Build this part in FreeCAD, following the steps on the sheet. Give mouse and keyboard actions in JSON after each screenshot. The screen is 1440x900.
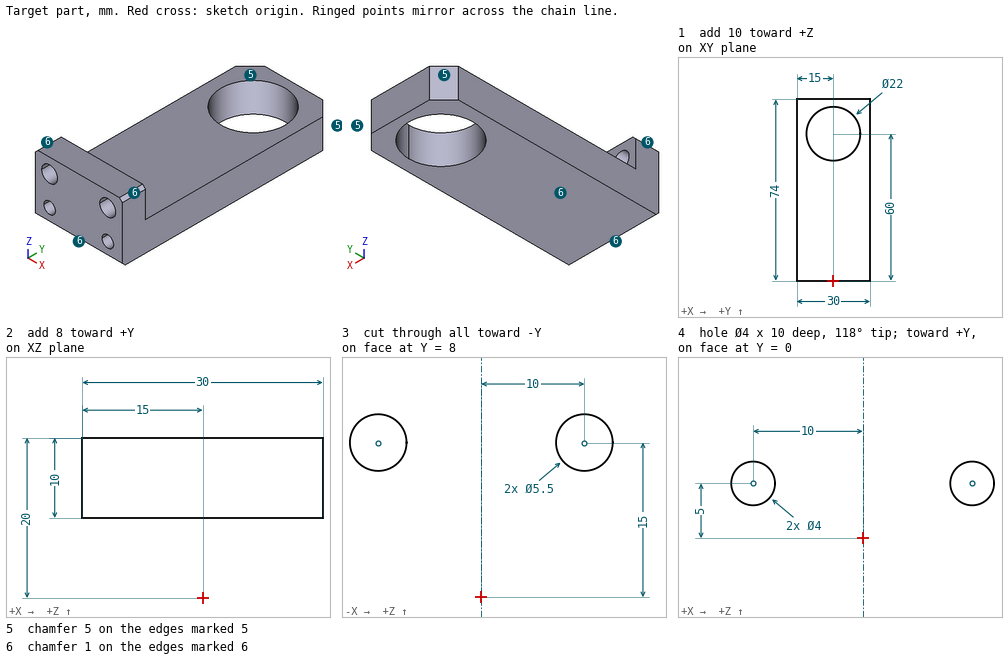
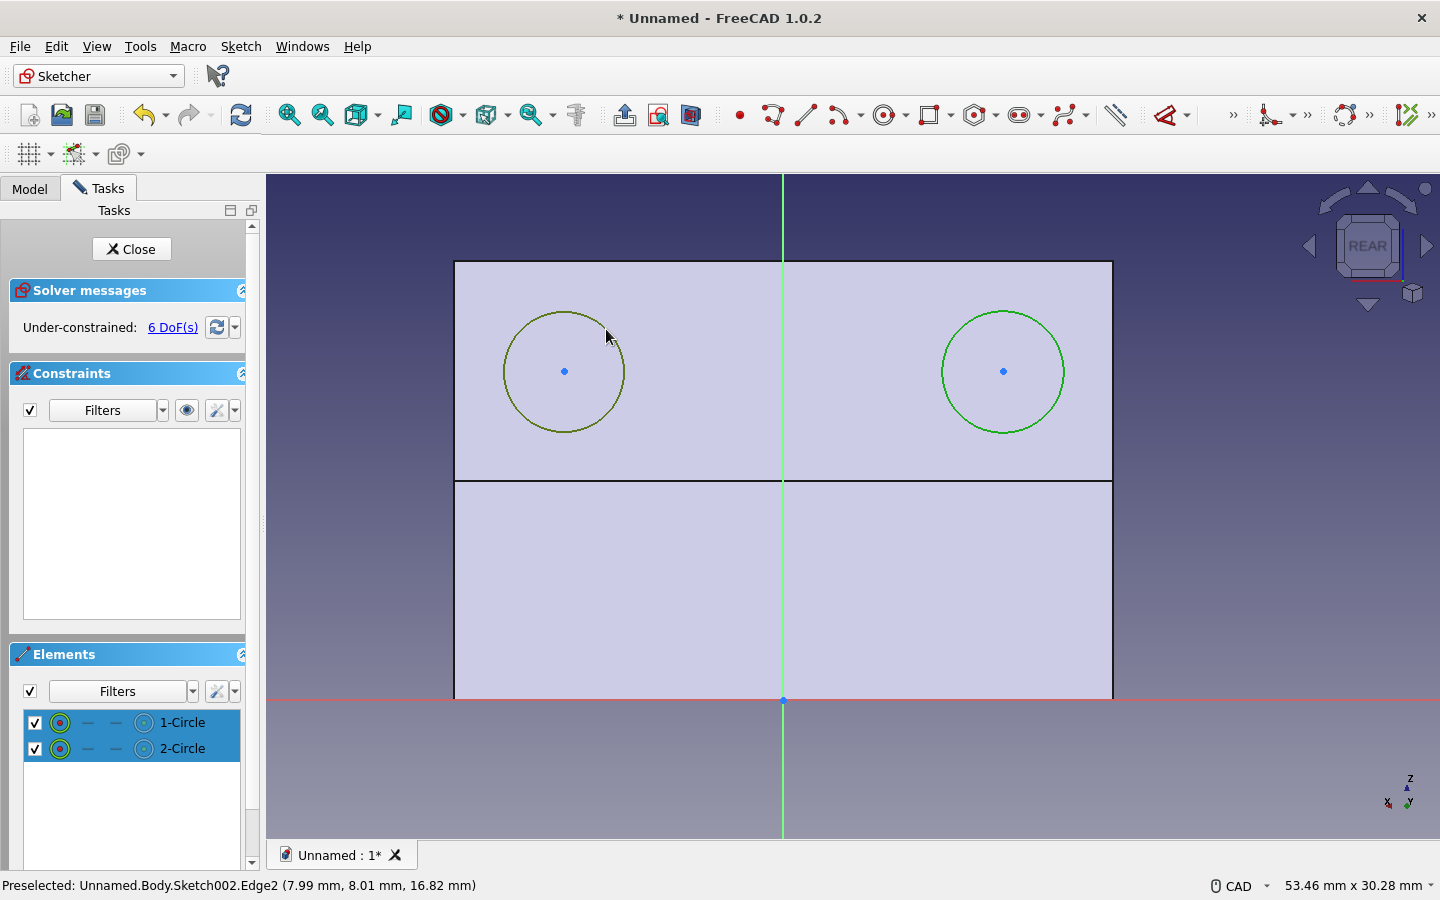
{"action": "key", "text": "e"}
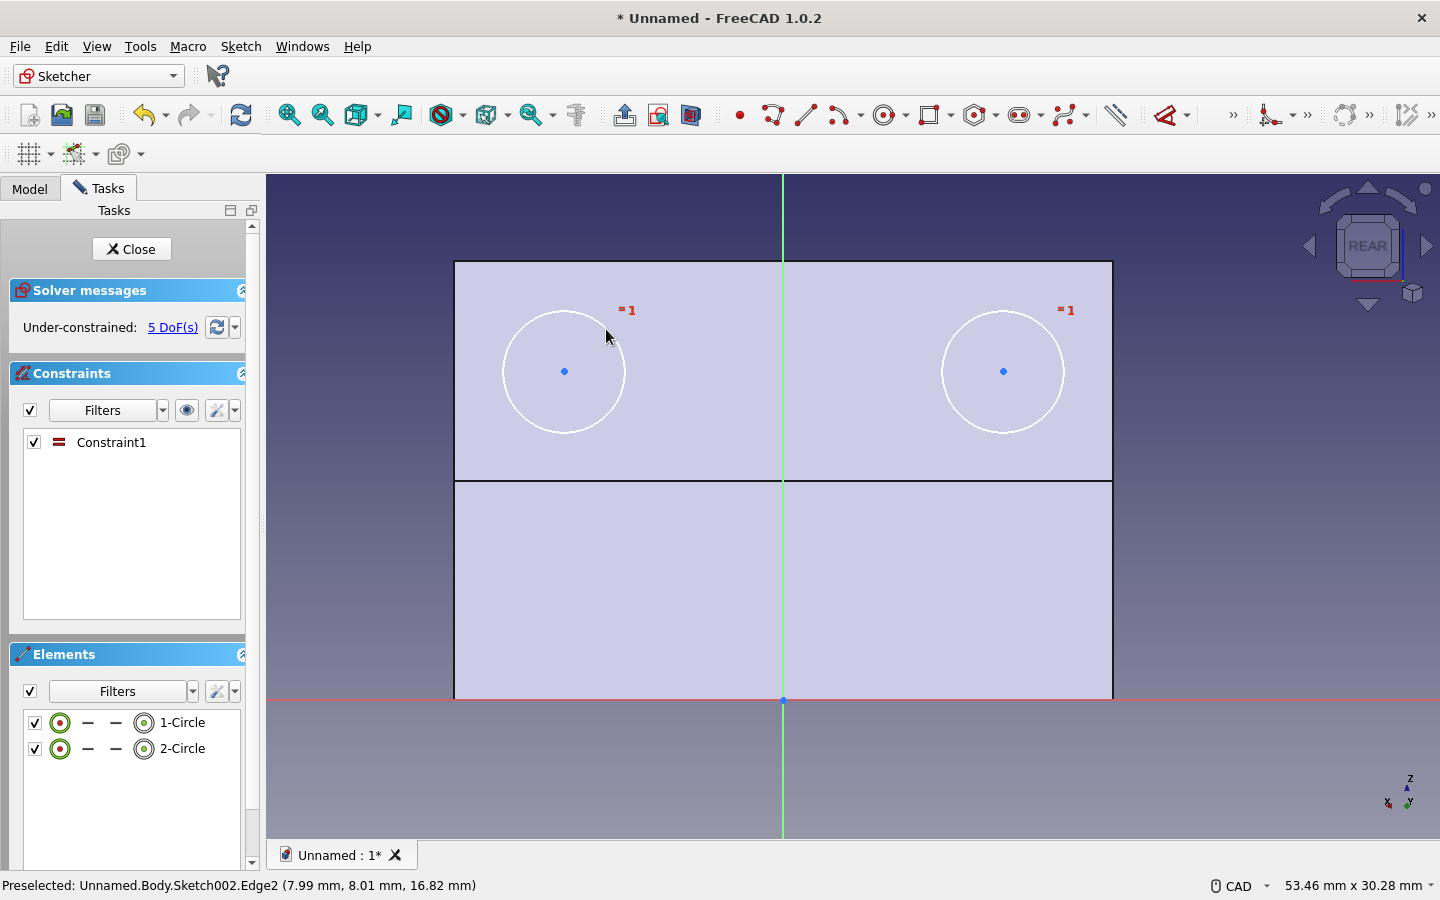
{"action": "left_click", "coordinate": [1003, 372]}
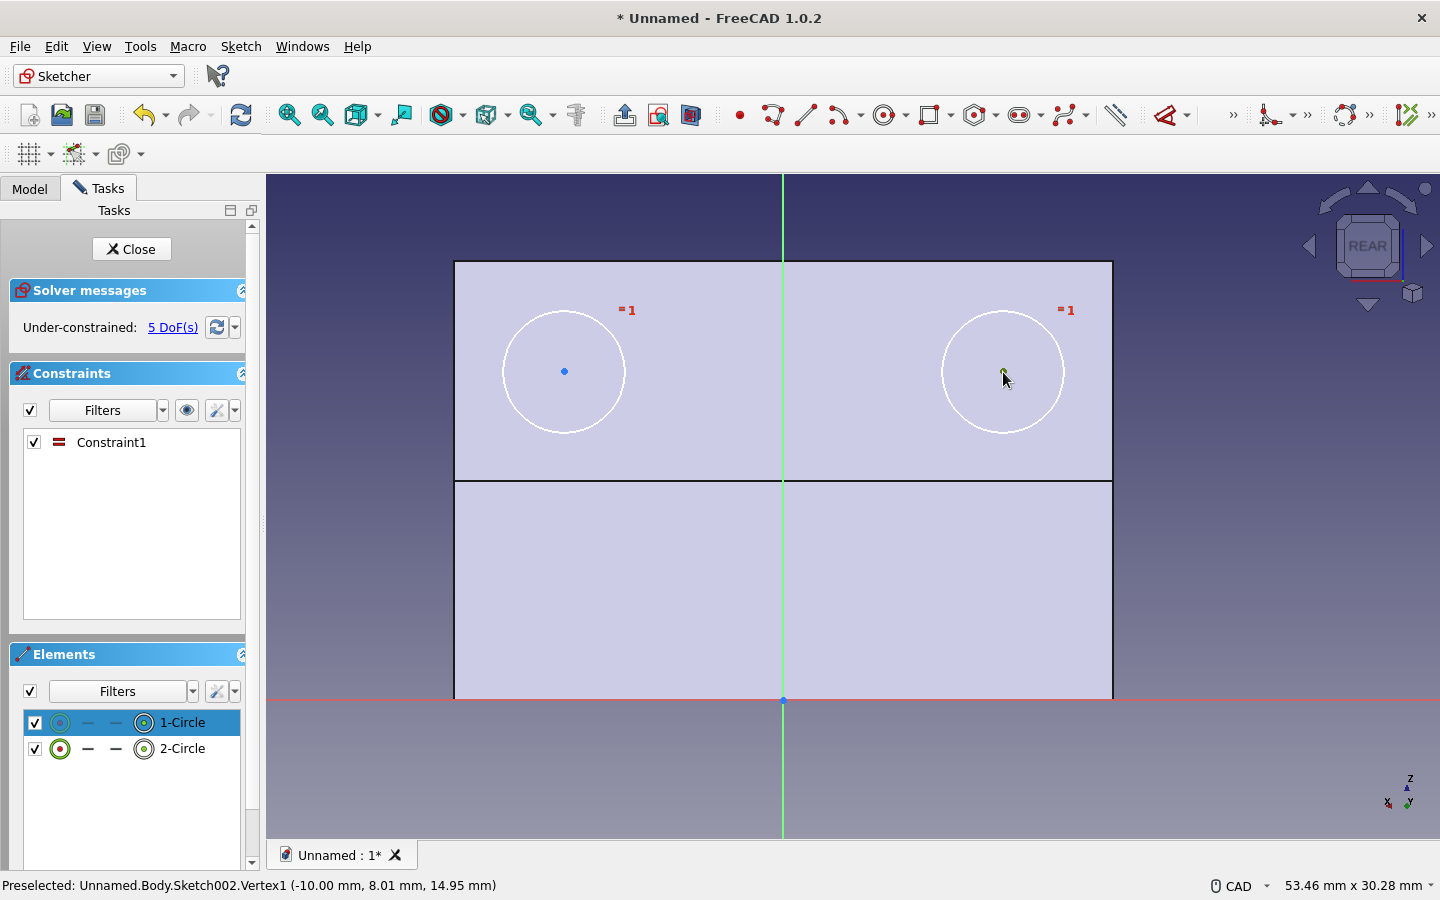
{"action": "left_click", "coordinate": [564, 372]}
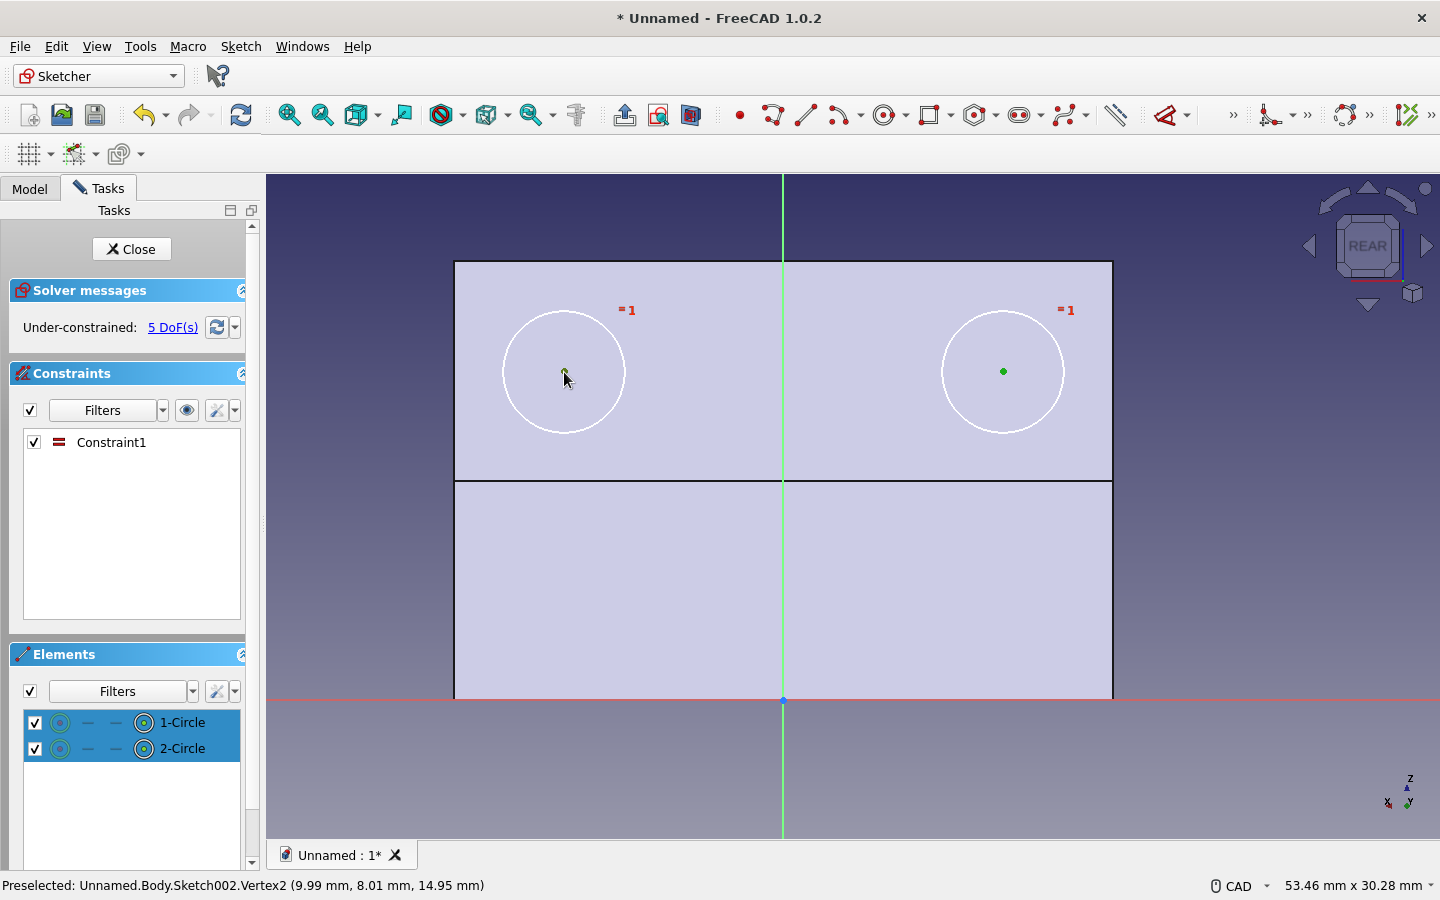
{"action": "left_click", "coordinate": [783, 768]}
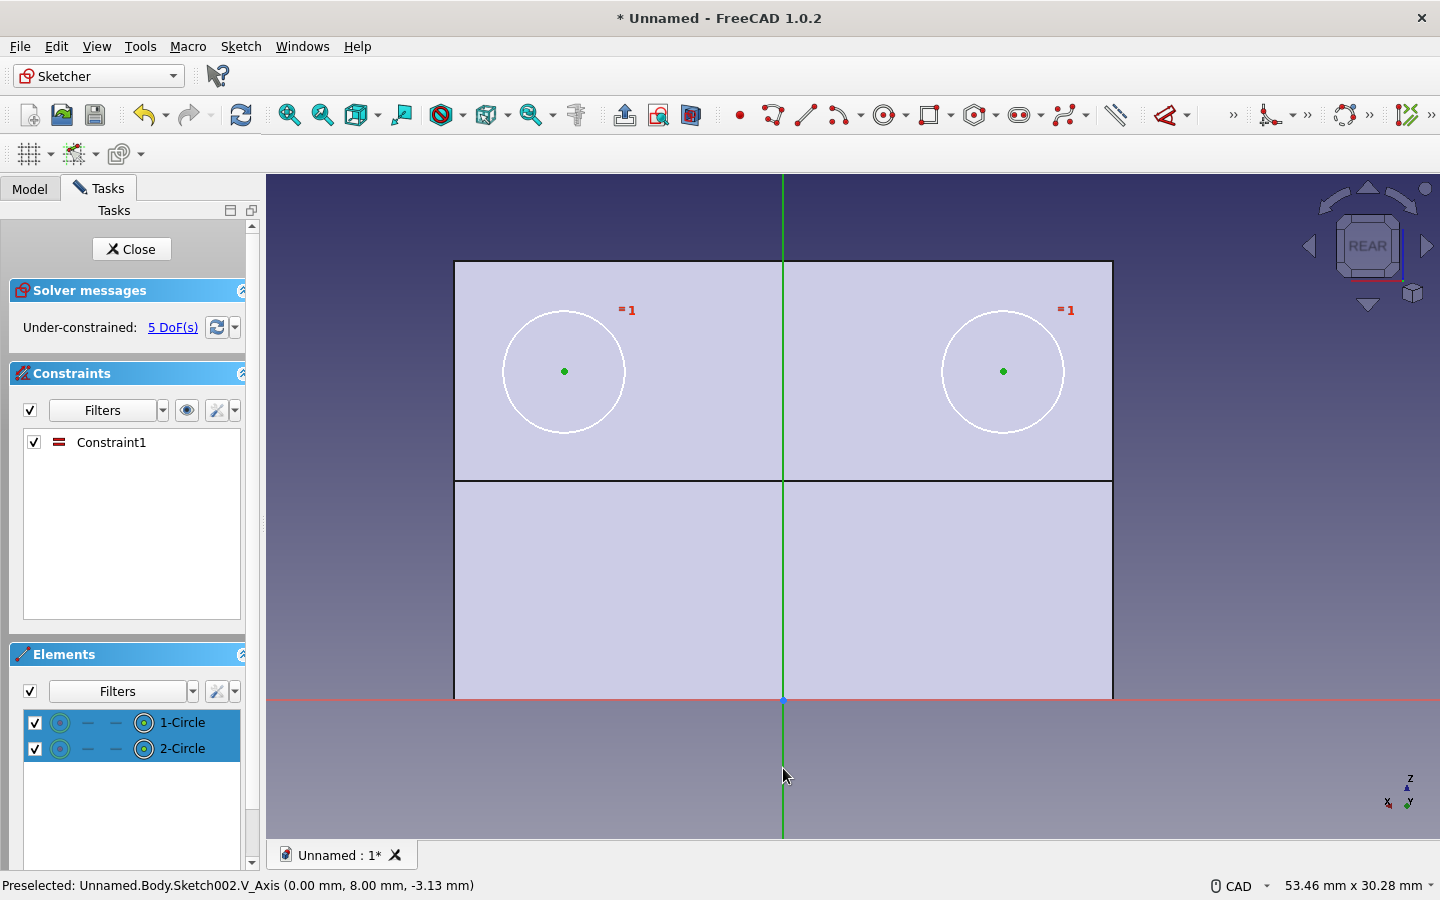
{"action": "key", "text": "s"}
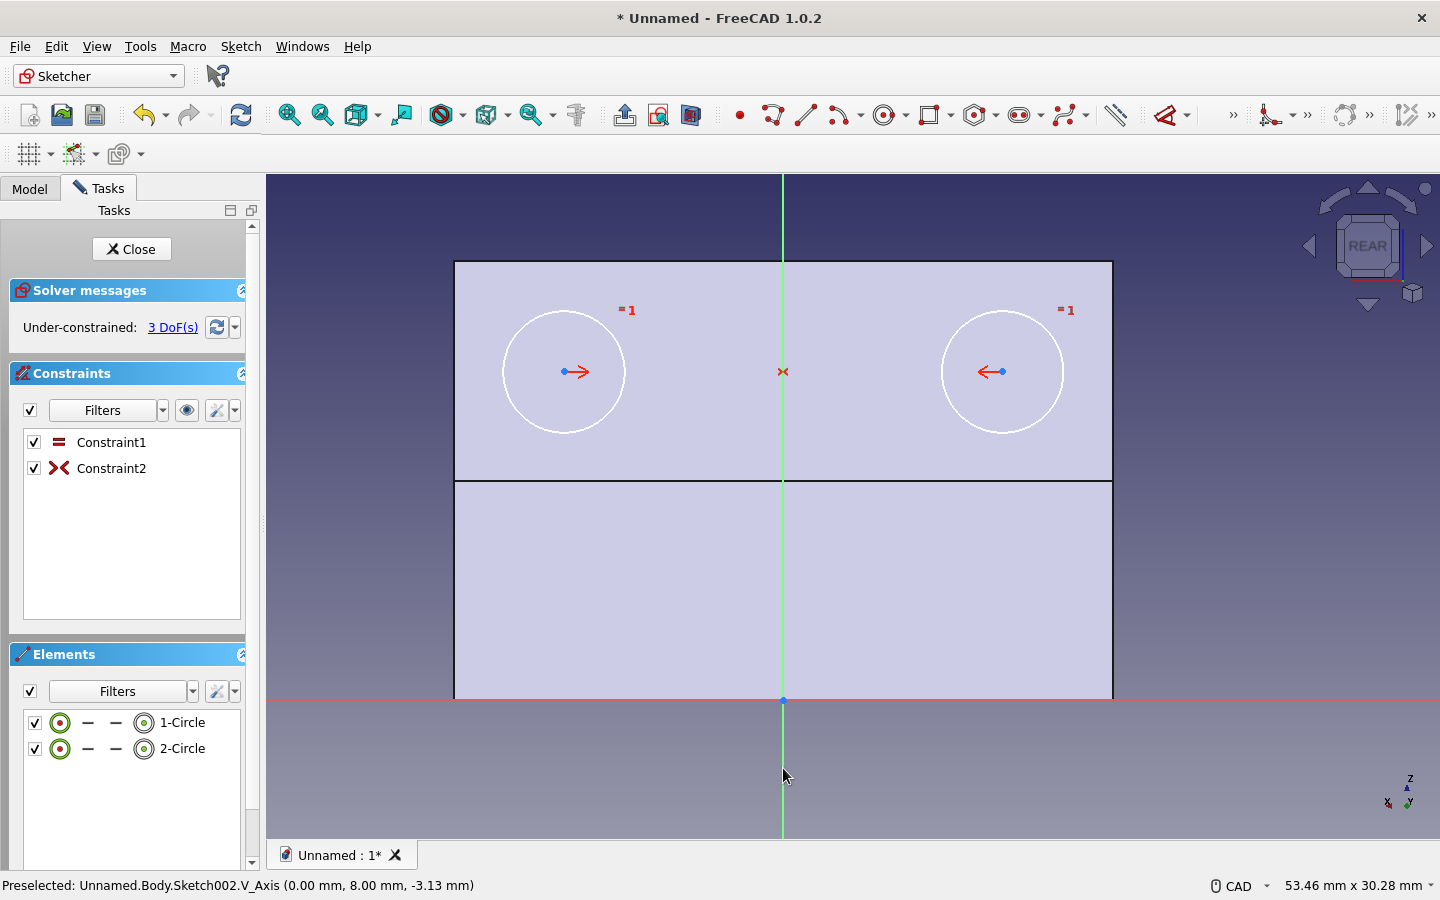
{"action": "left_click", "coordinate": [1164, 116]}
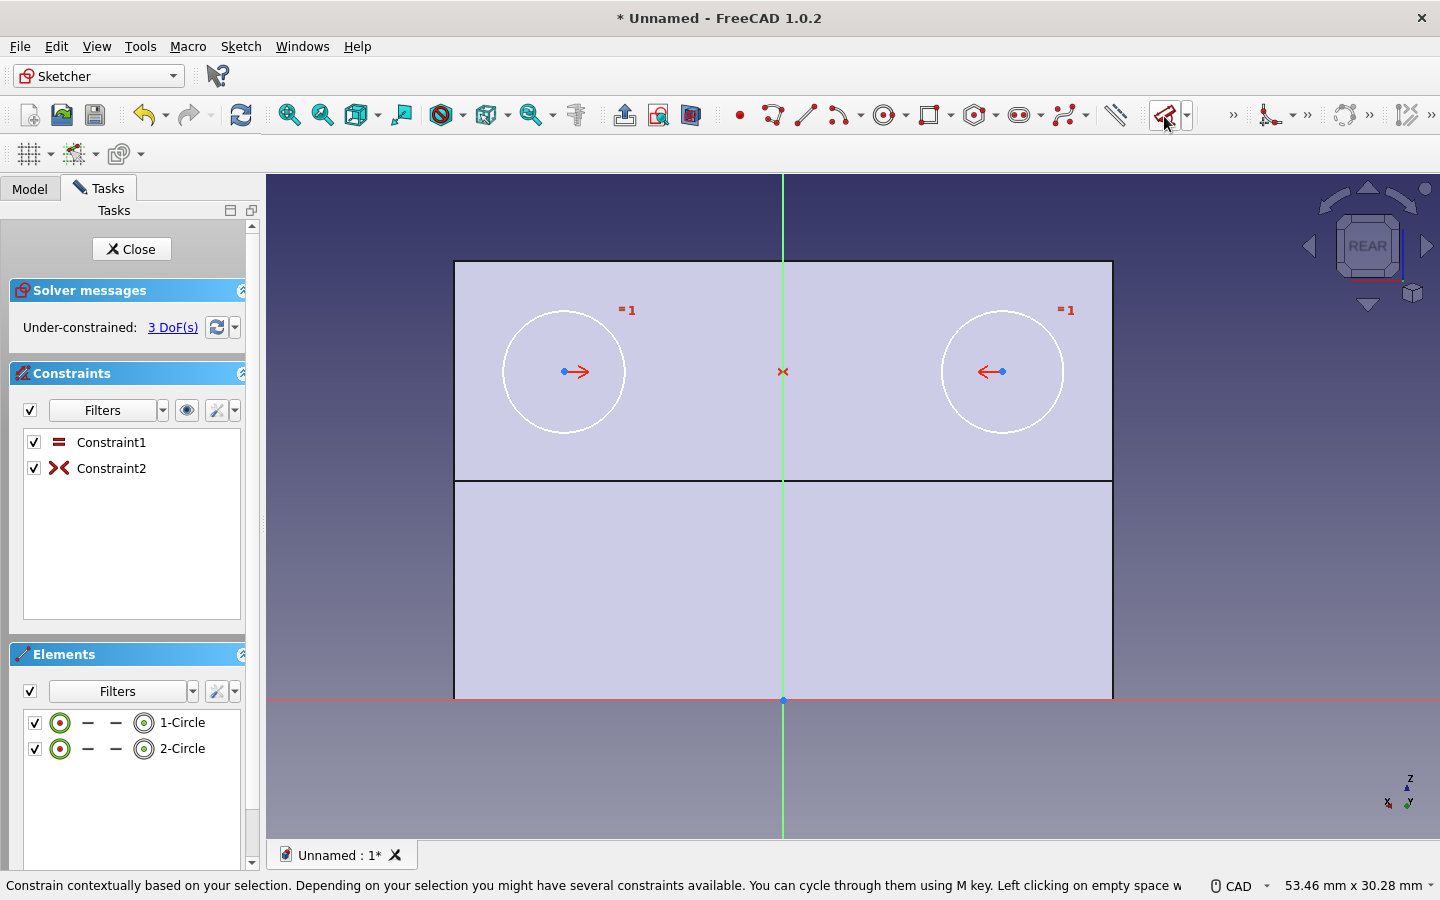
{"action": "left_click", "coordinate": [1046, 329]}
{"action": "left_click", "coordinate": [1069, 306]}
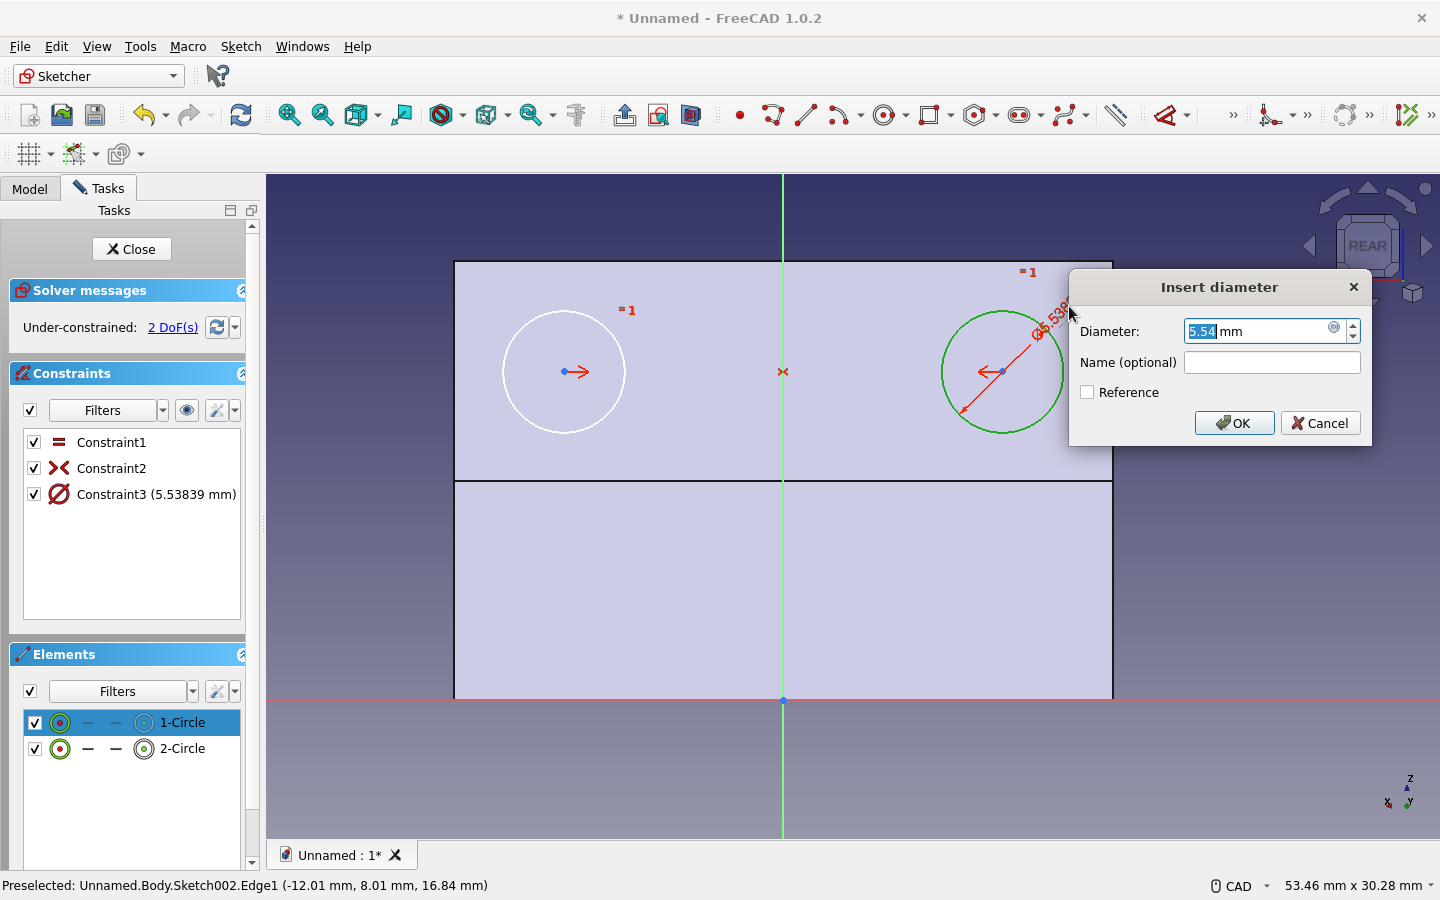
{"action": "type", "text": "5.5"}
{"action": "key", "text": "Return"}